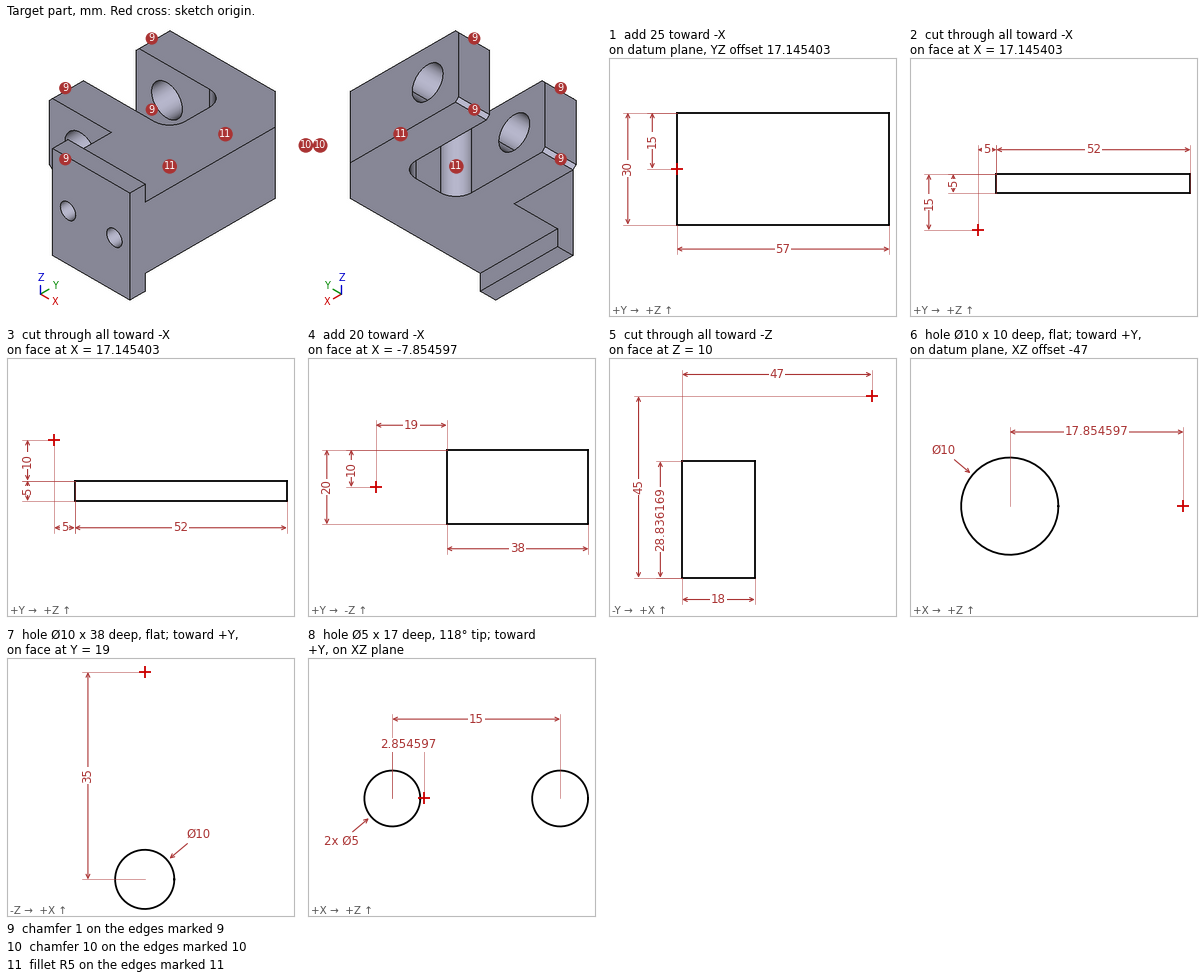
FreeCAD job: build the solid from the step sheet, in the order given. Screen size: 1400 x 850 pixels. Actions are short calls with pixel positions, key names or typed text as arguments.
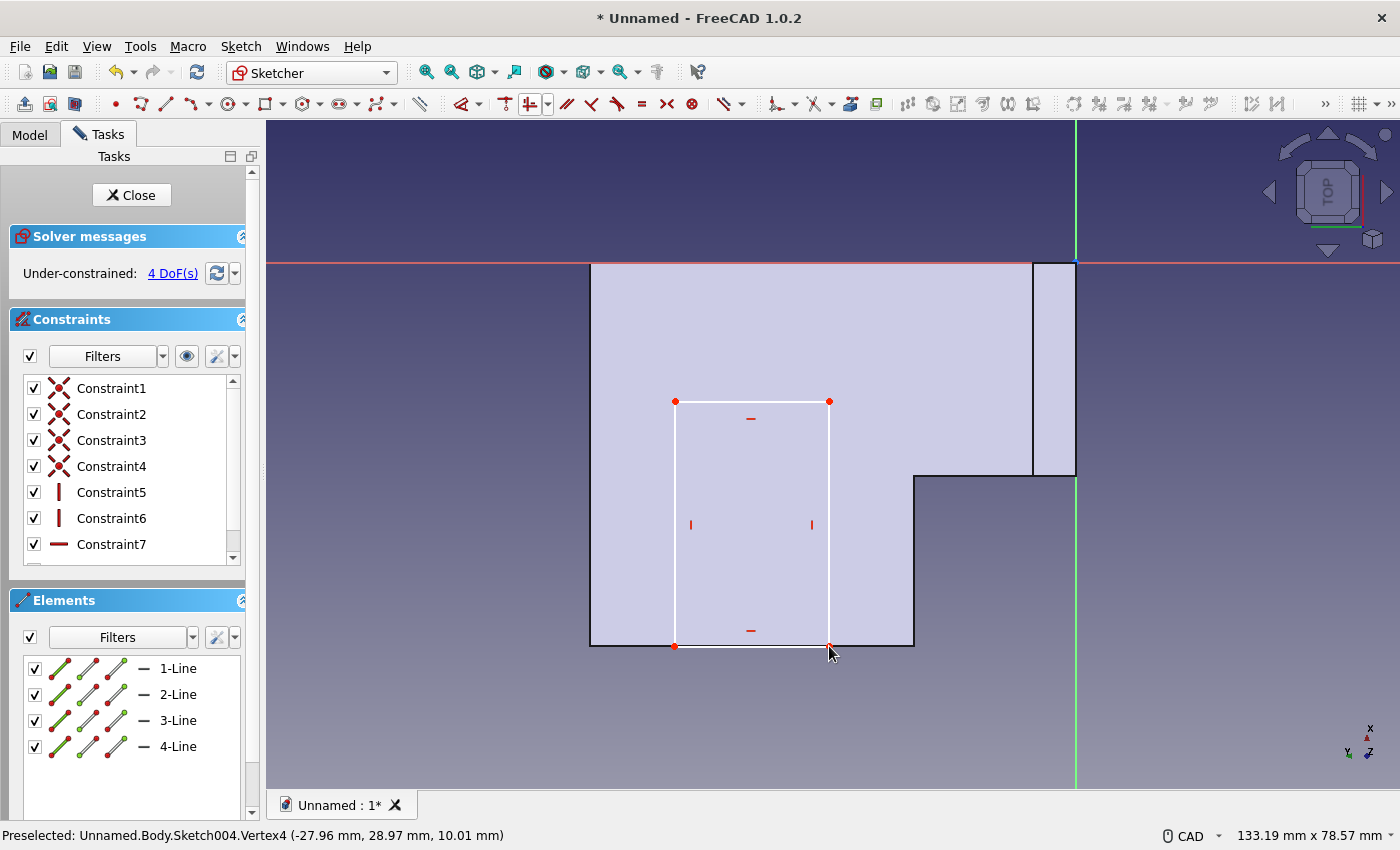
click(460, 104)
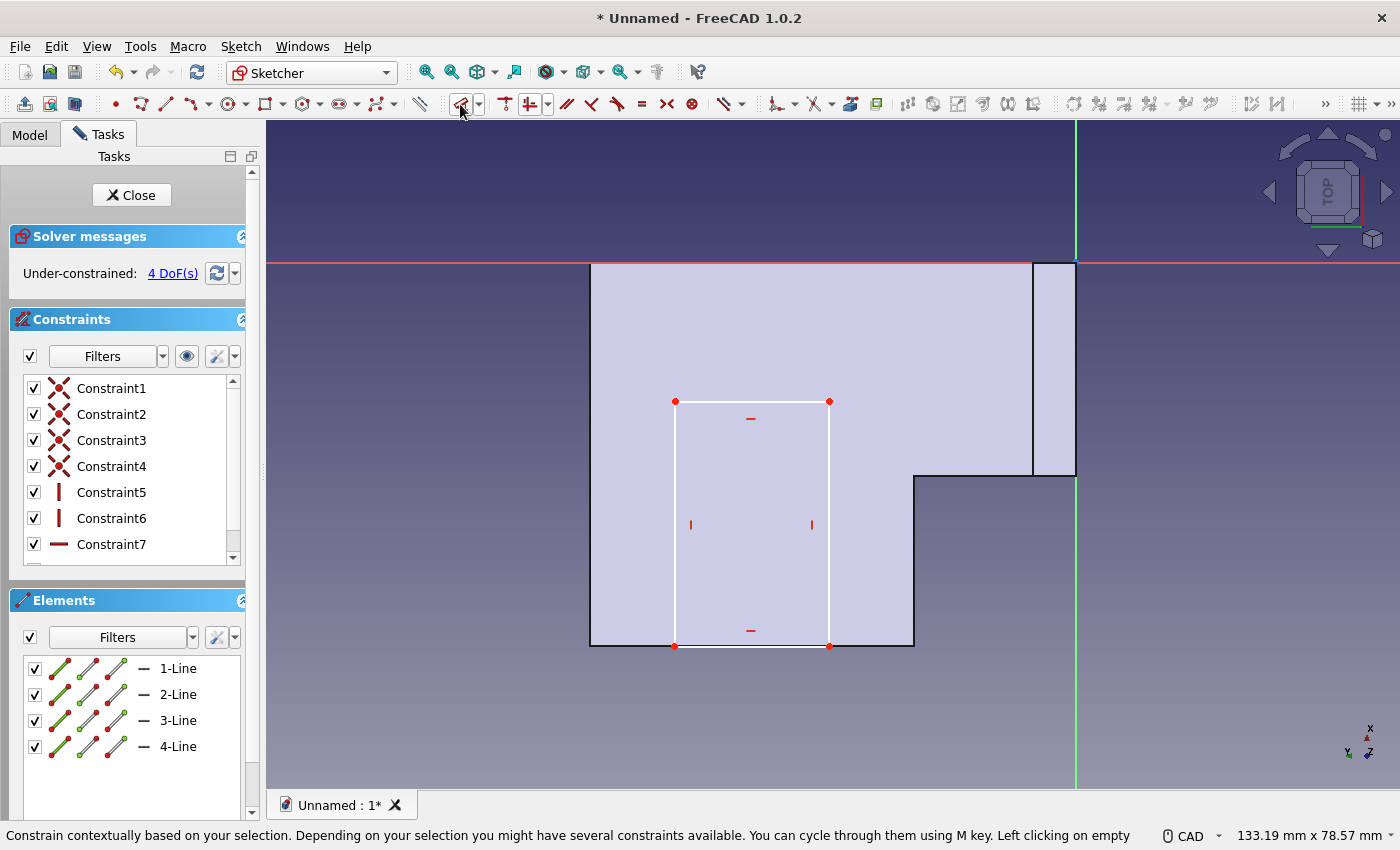
click(721, 647)
click(752, 681)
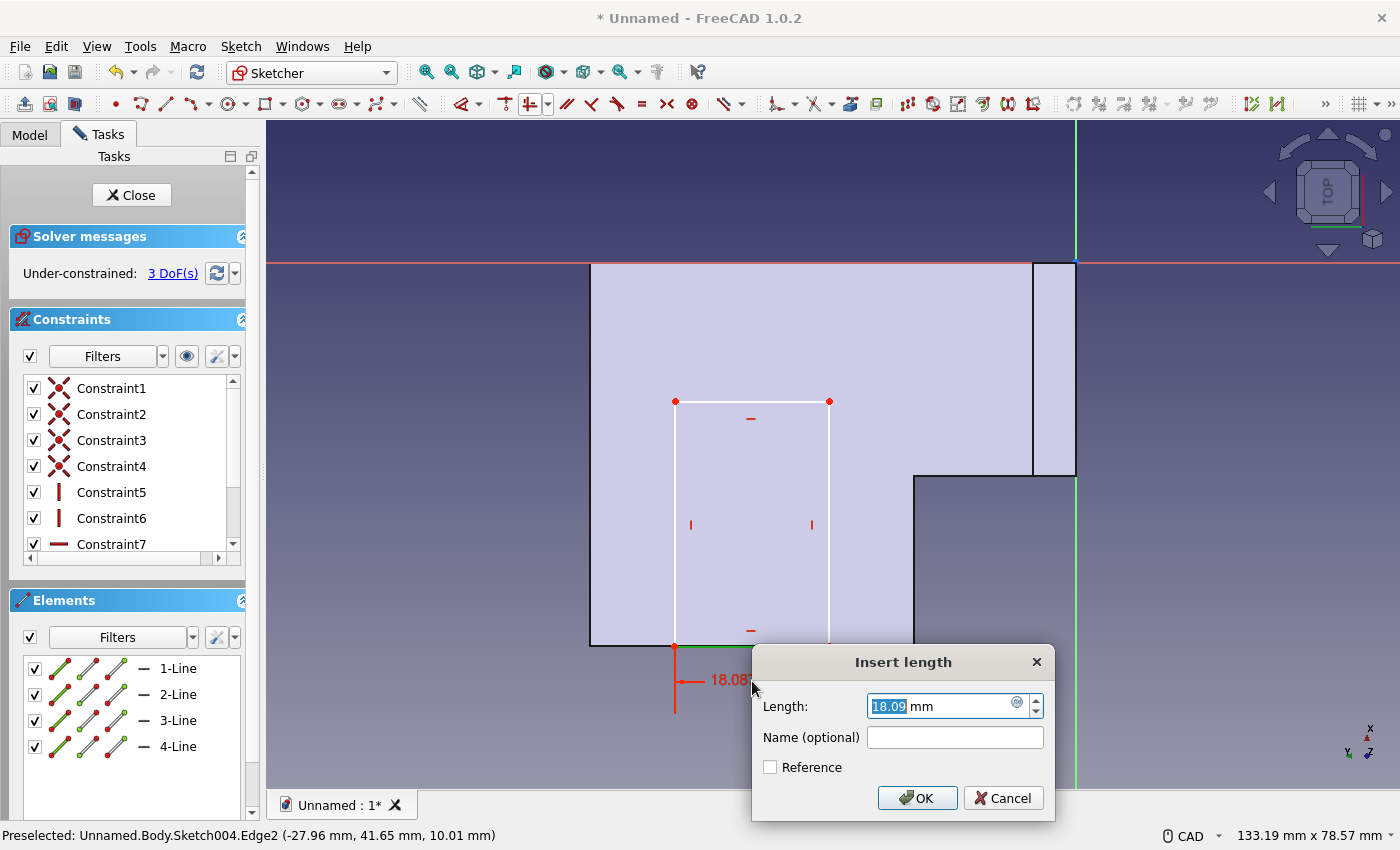
text(18)
key(Return)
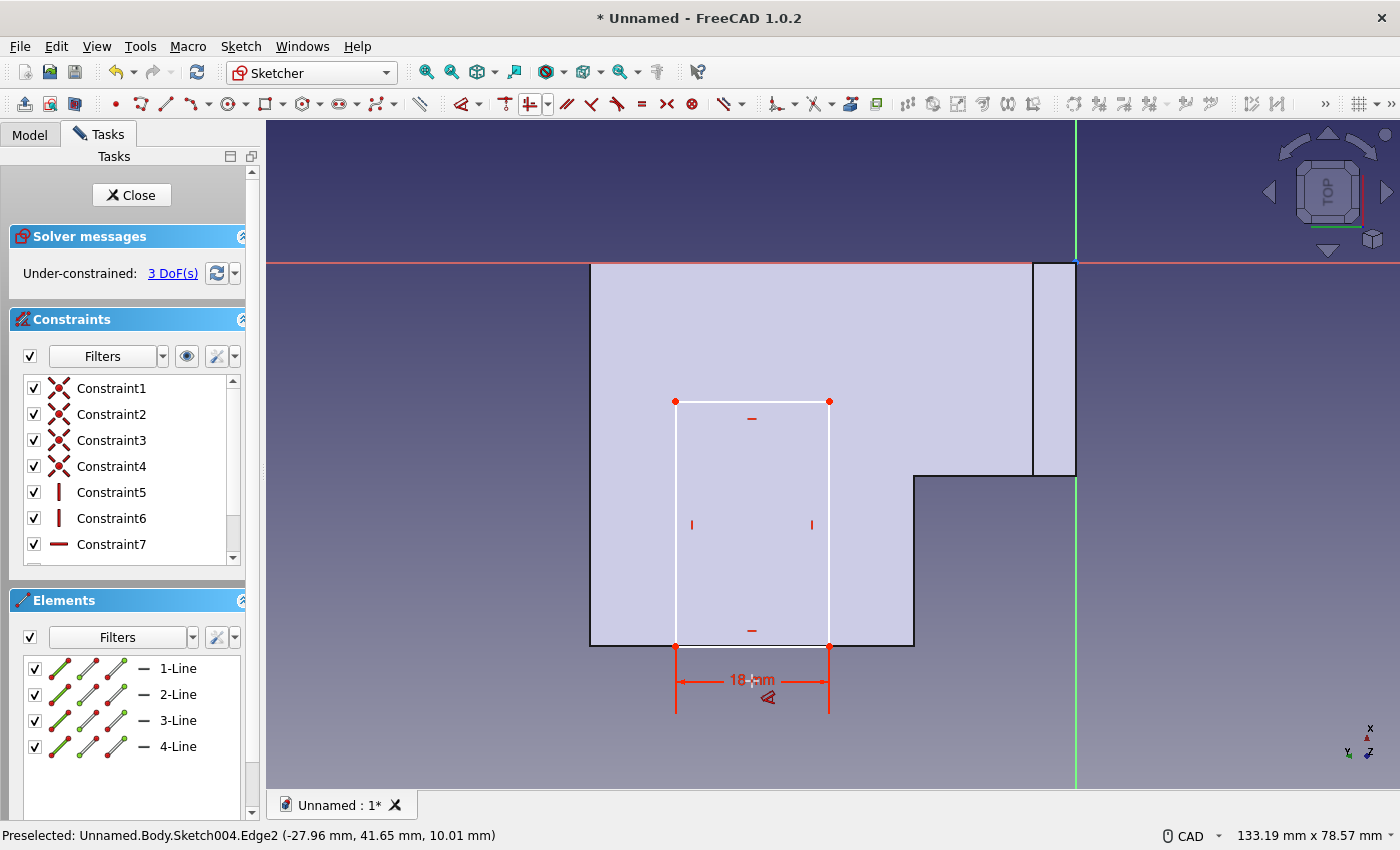
click(676, 402)
click(876, 229)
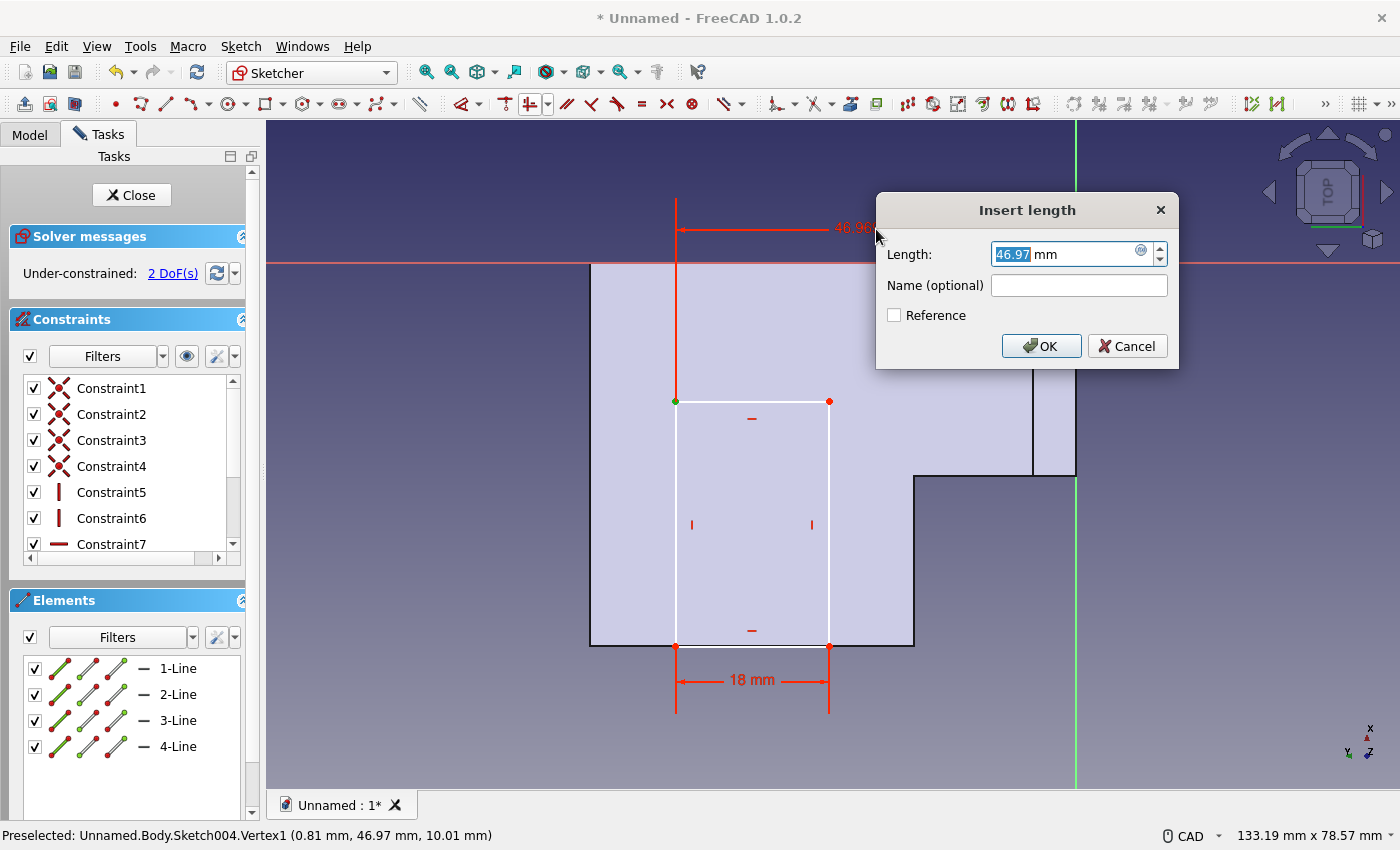
text(47)
key(Return)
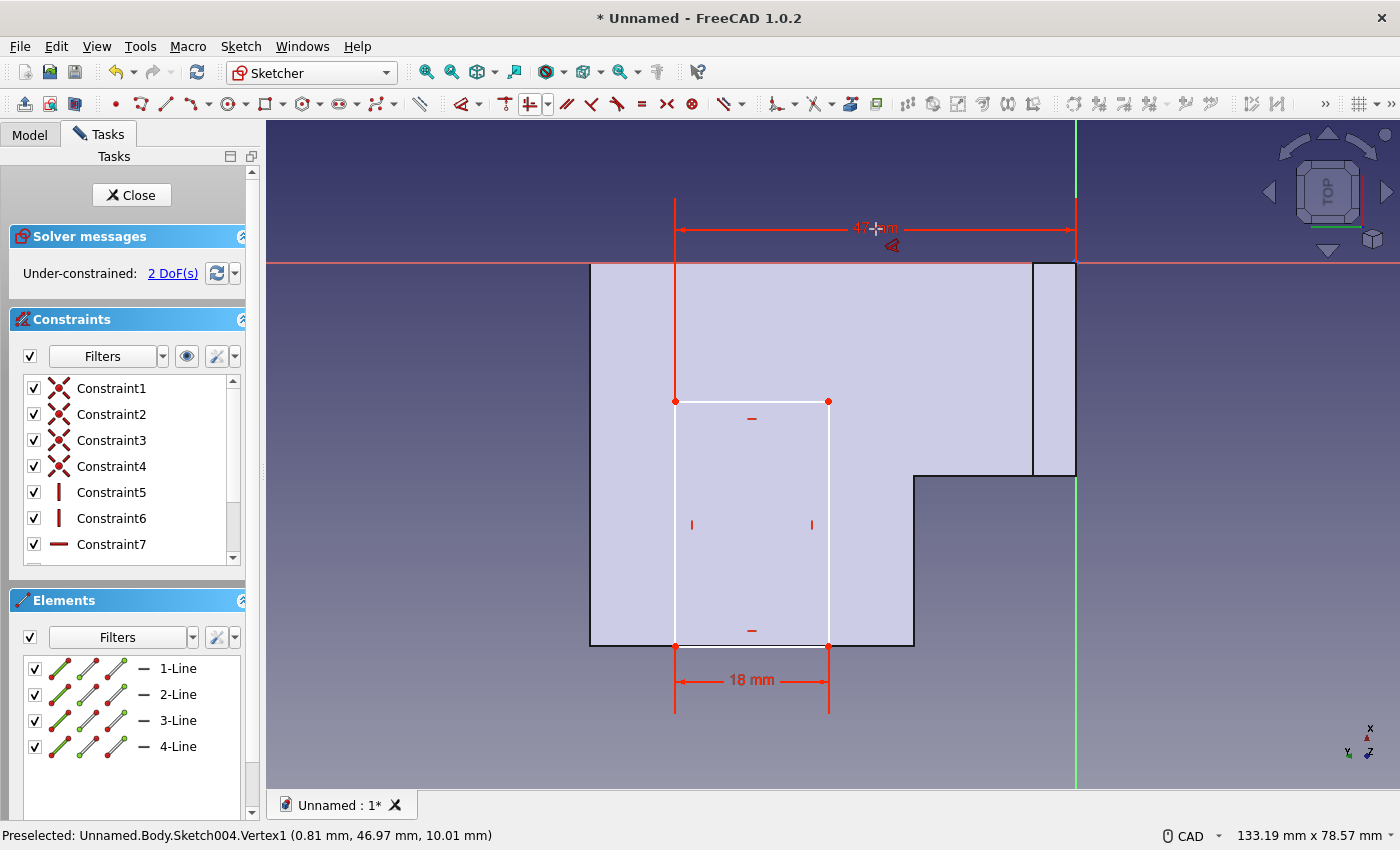
click(675, 647)
click(1110, 455)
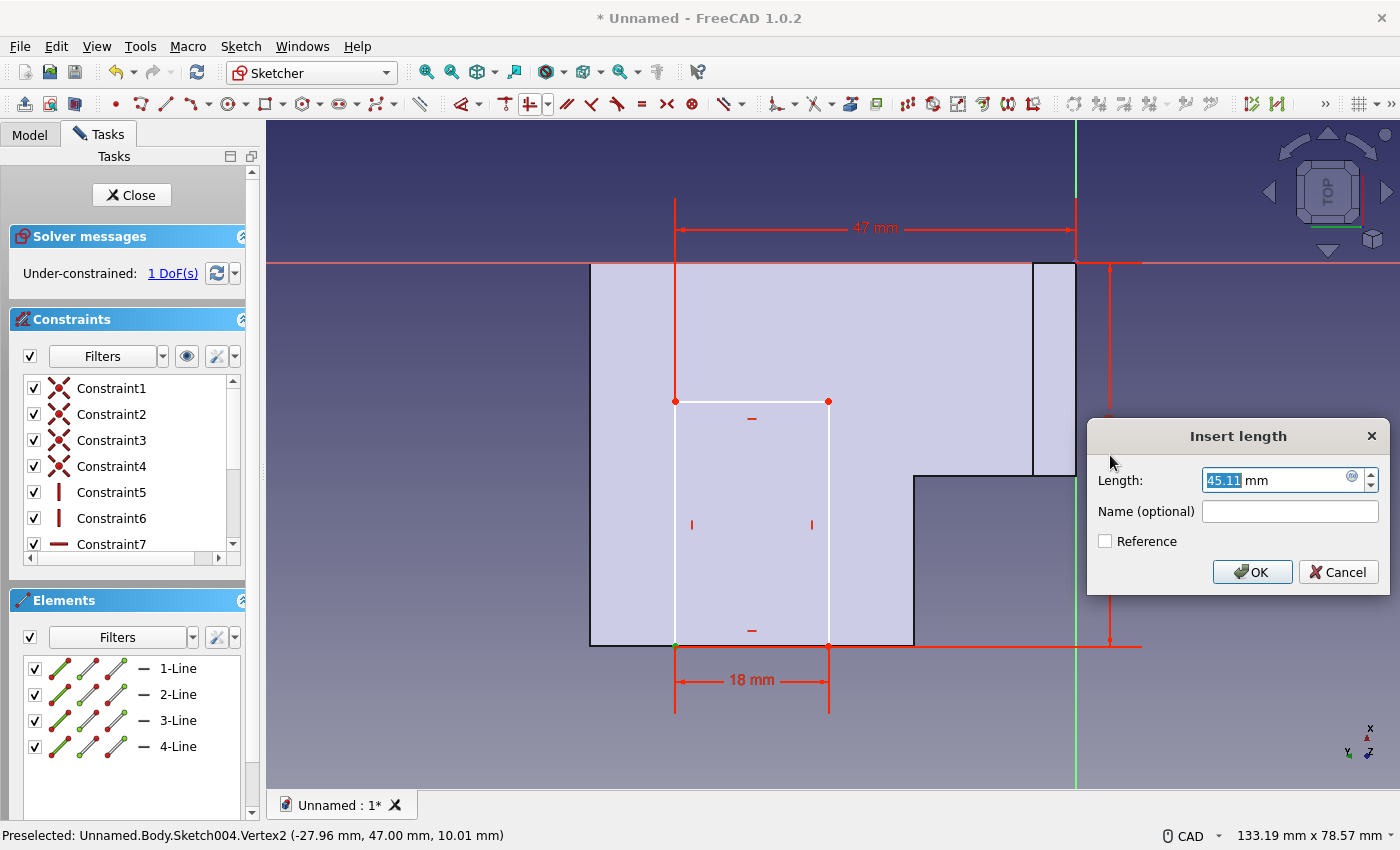
text(45)
key(Return)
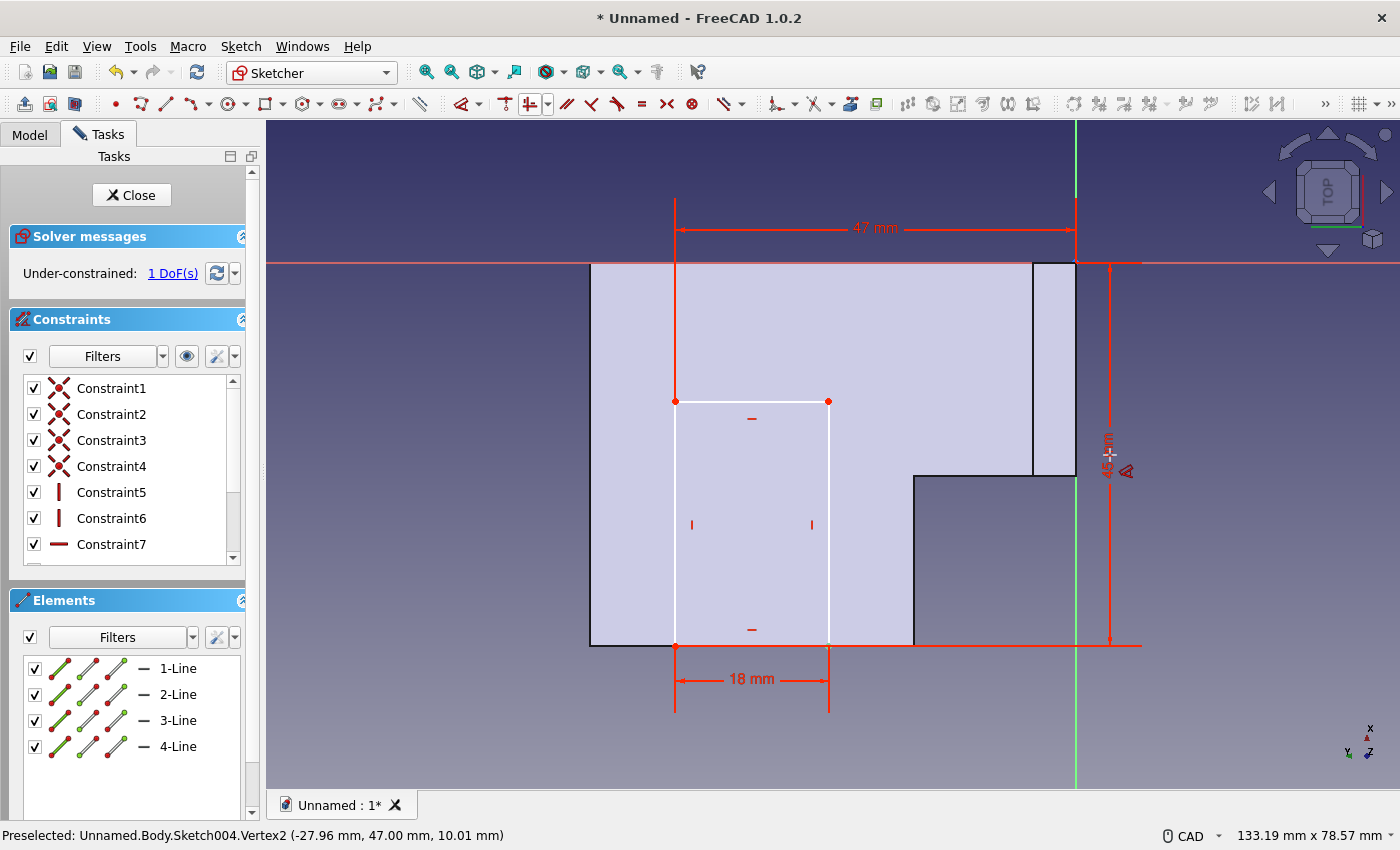
click(675, 475)
click(641, 524)